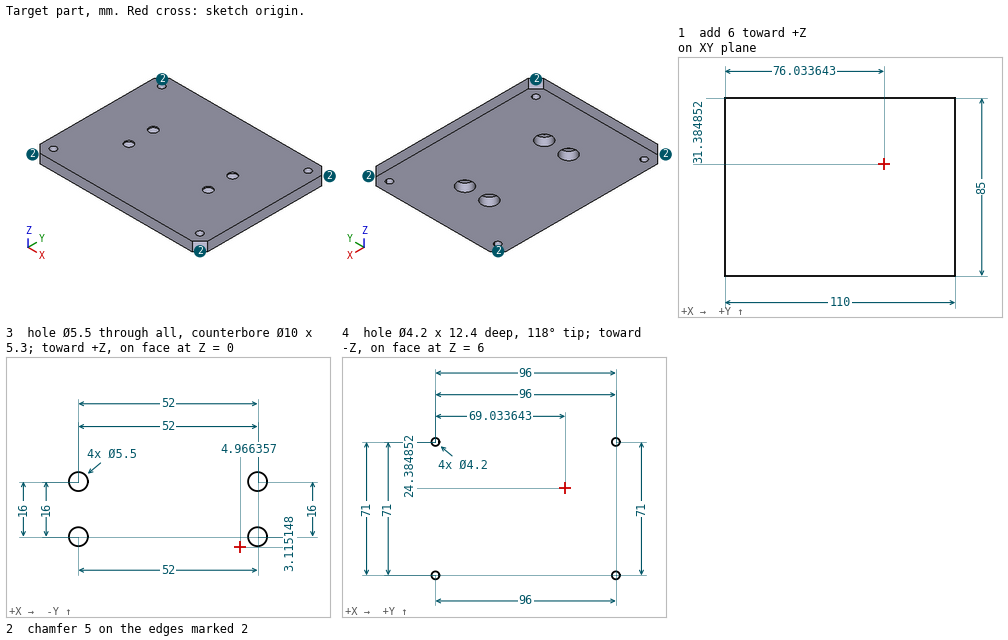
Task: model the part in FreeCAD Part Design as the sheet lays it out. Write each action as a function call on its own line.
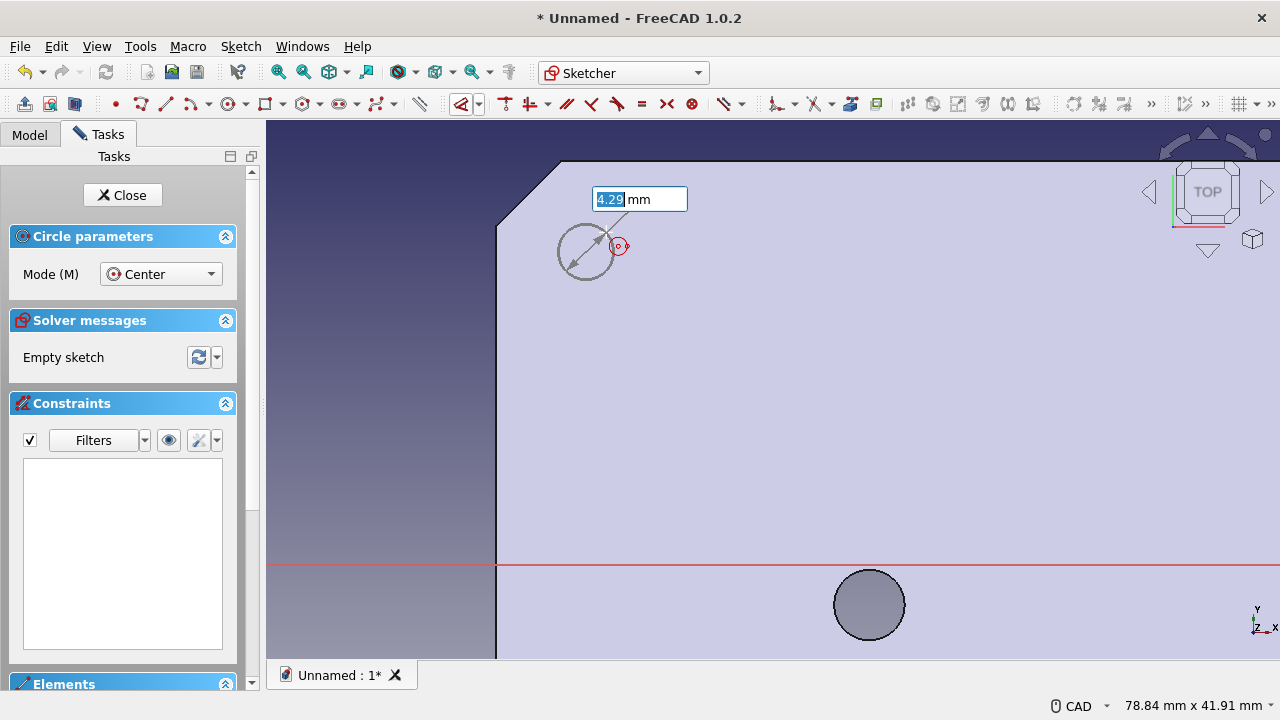
text(4.2)
key(Return)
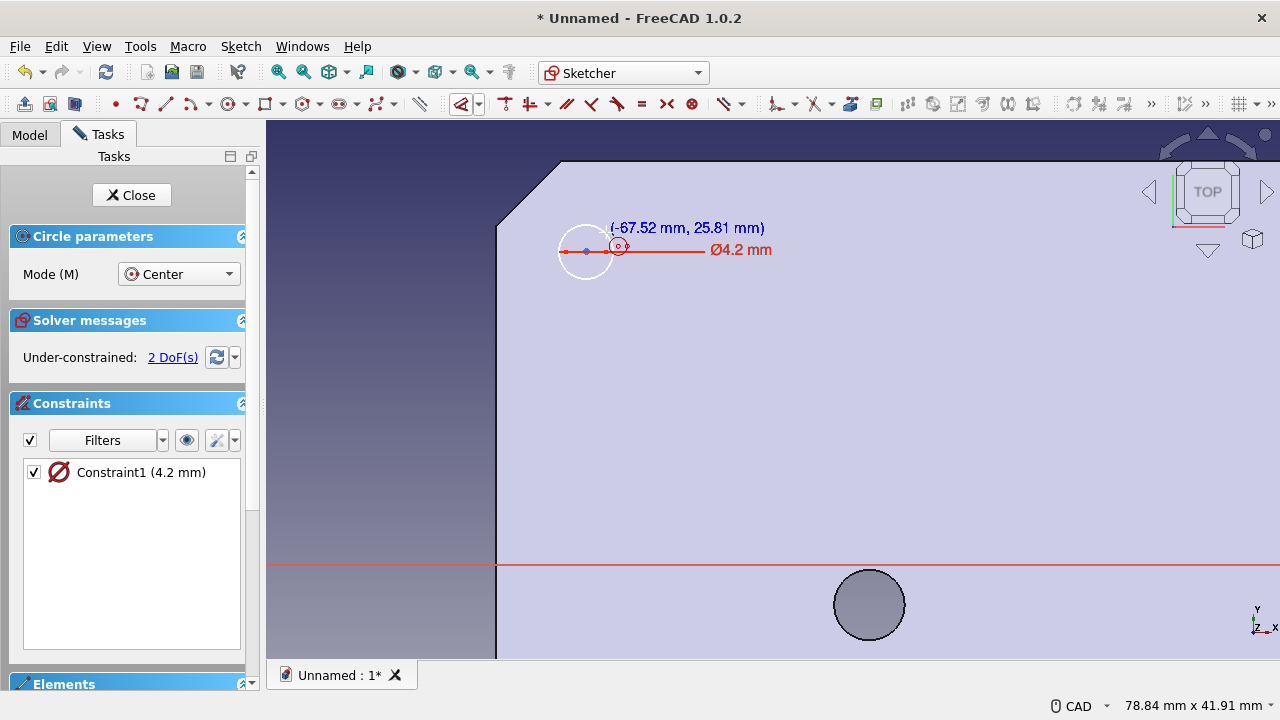
scroll(414, 204, down, 5)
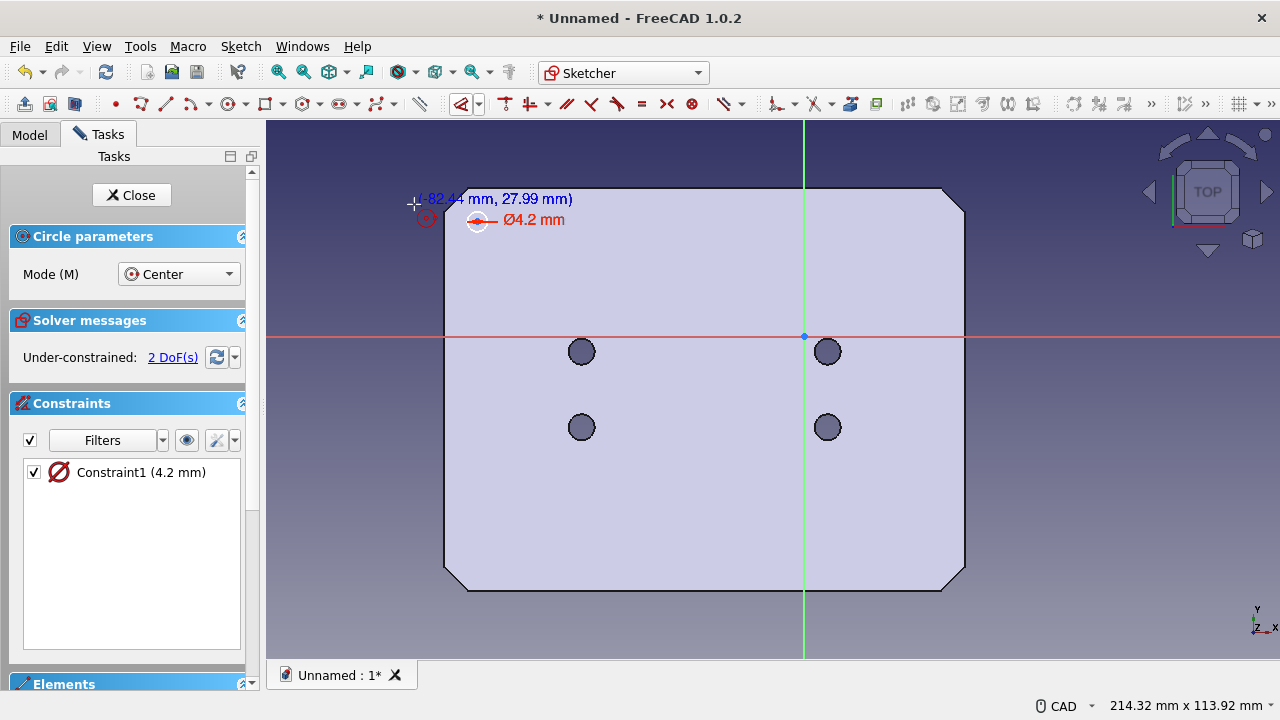
scroll(932, 222, up, 5)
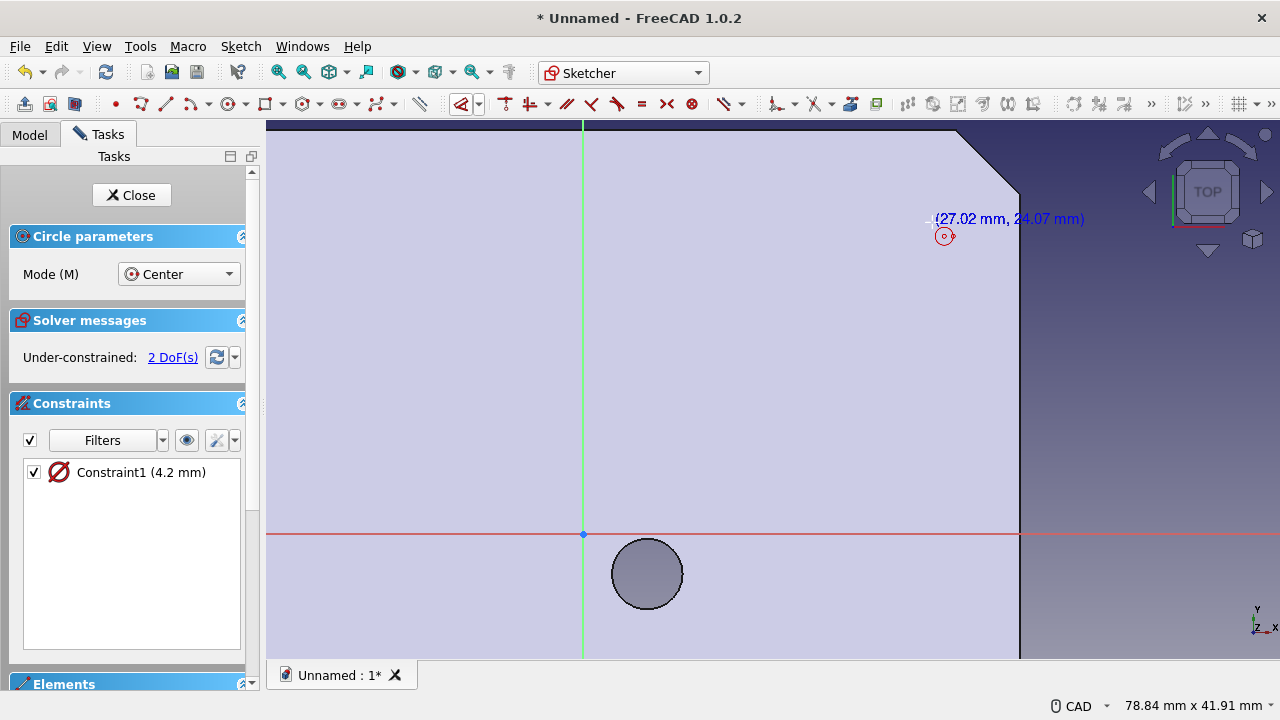
click(930, 220)
move(949, 201)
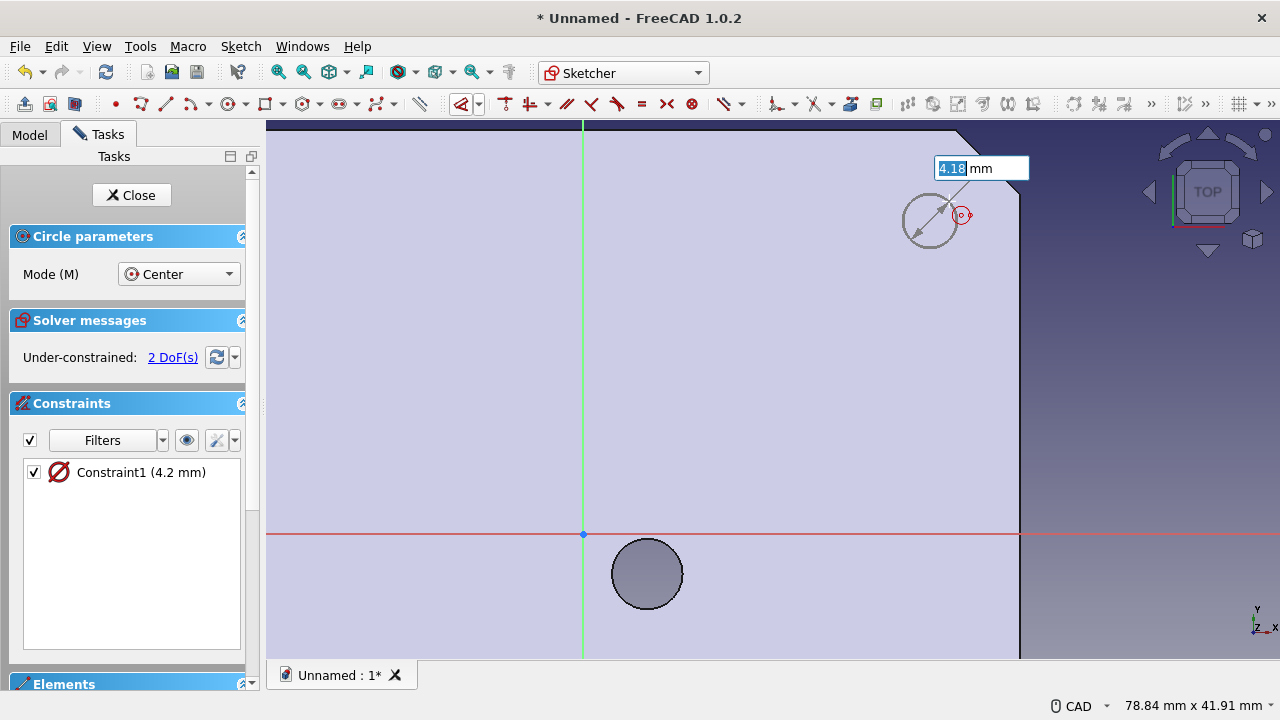
text(4.2)
key(Return)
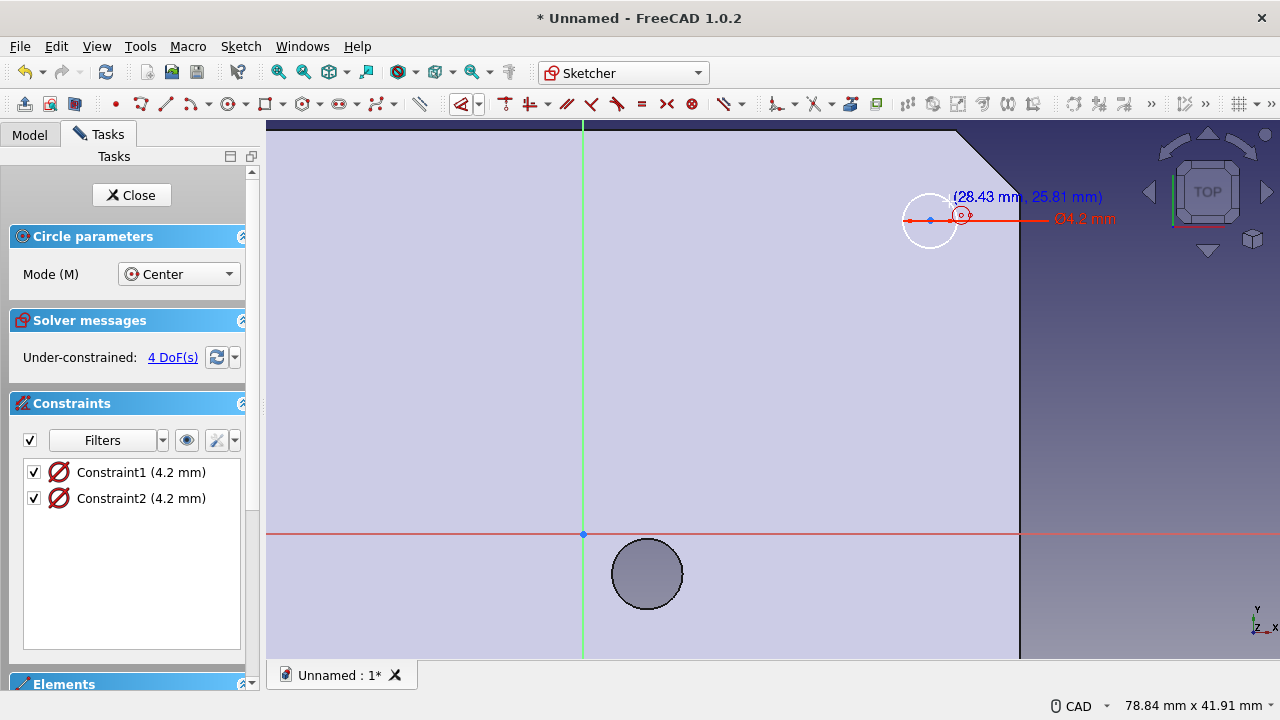
scroll(932, 222, down, 5)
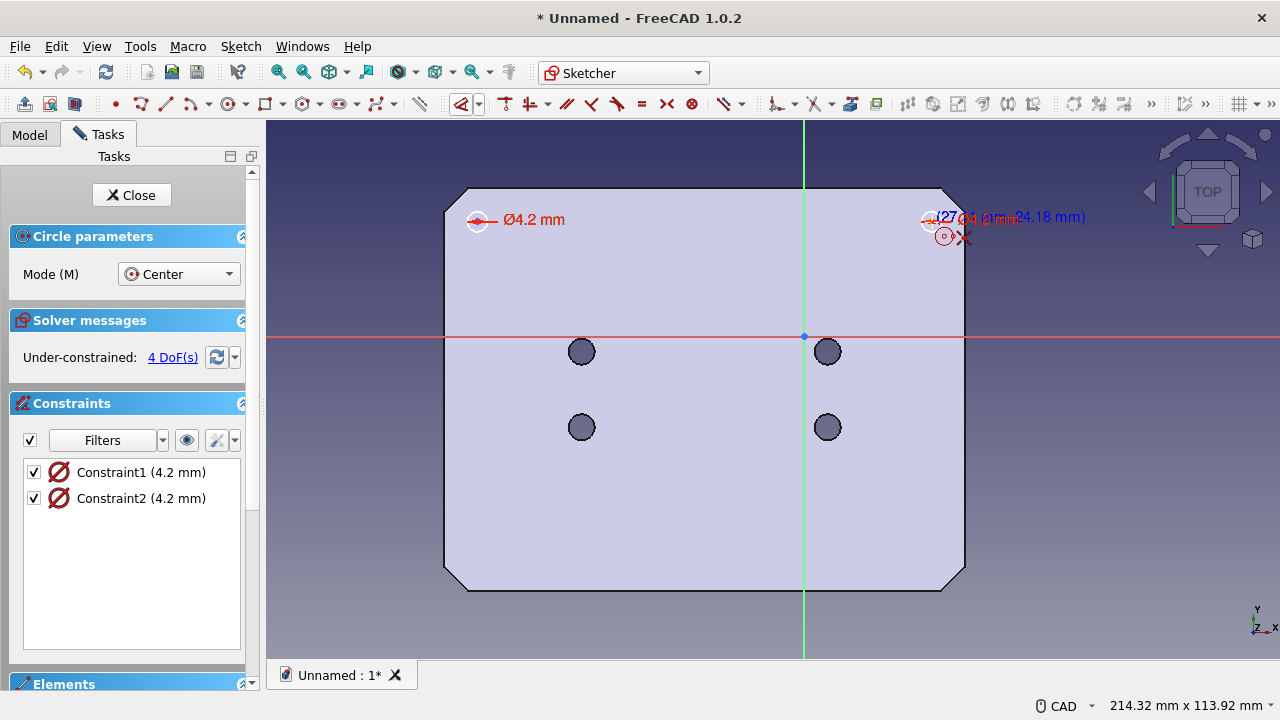
scroll(932, 557, up, 5)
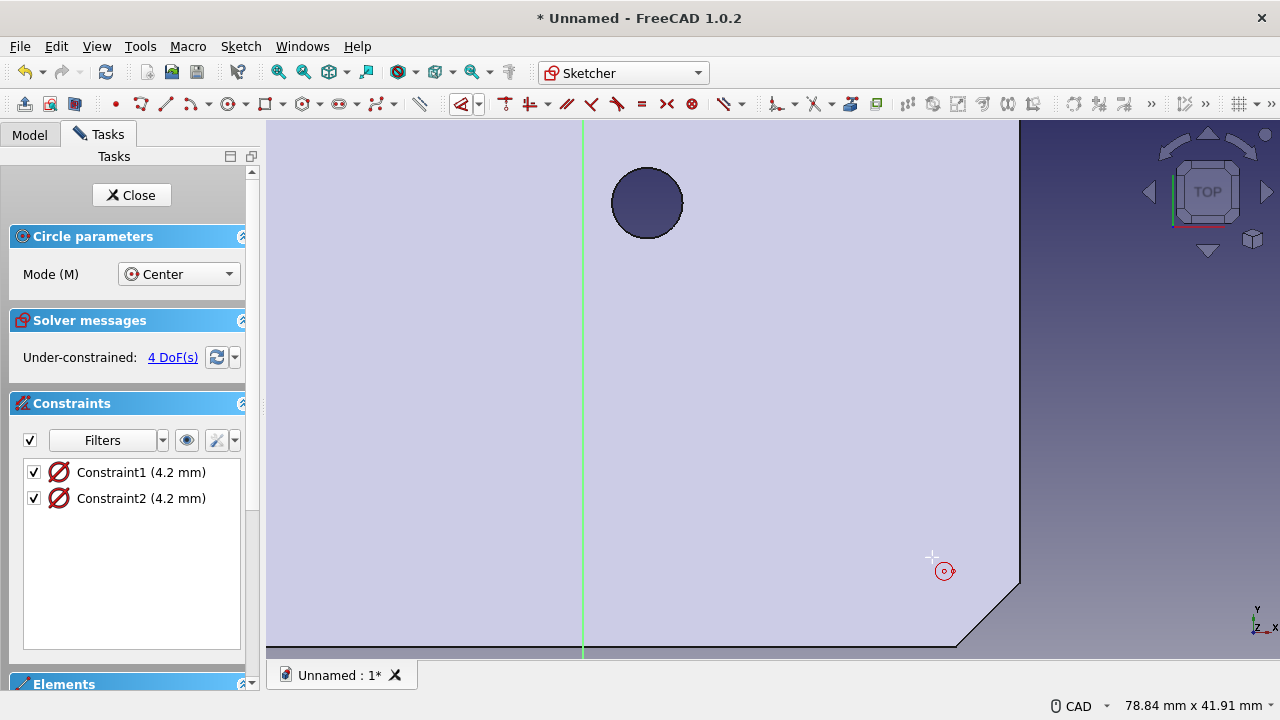
click(930, 557)
move(949, 538)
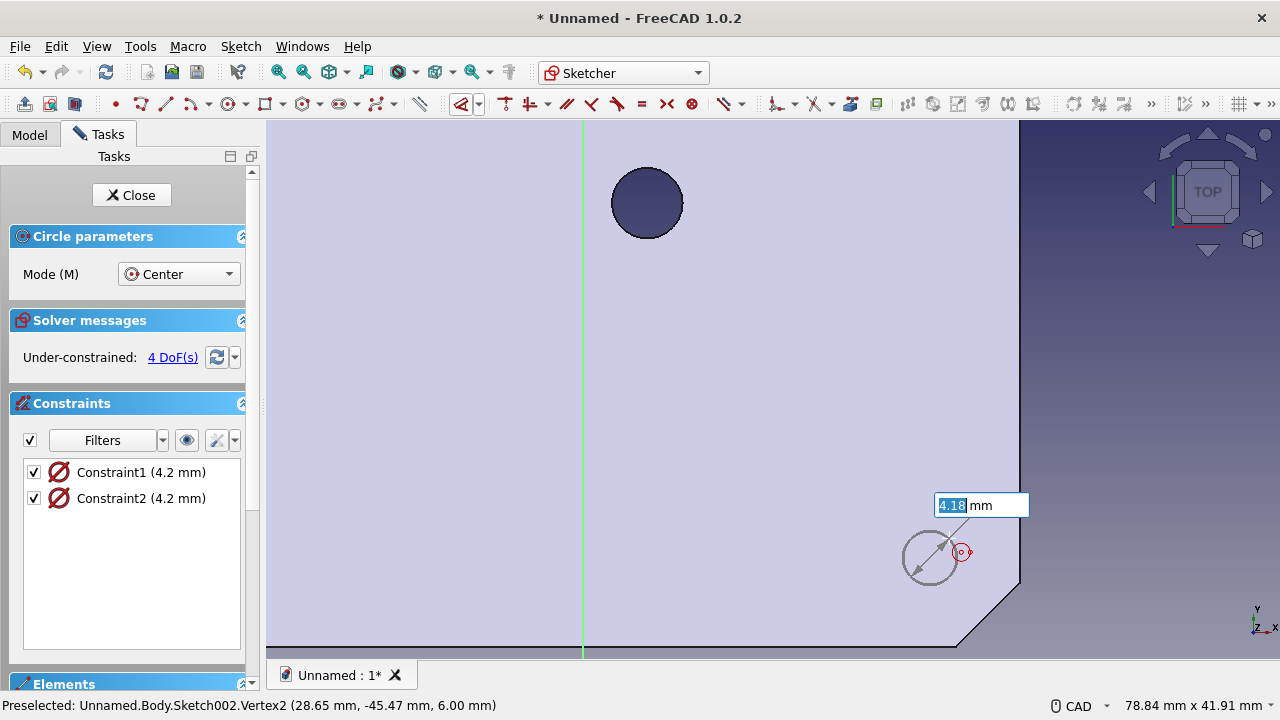
text(4.2)
key(Return)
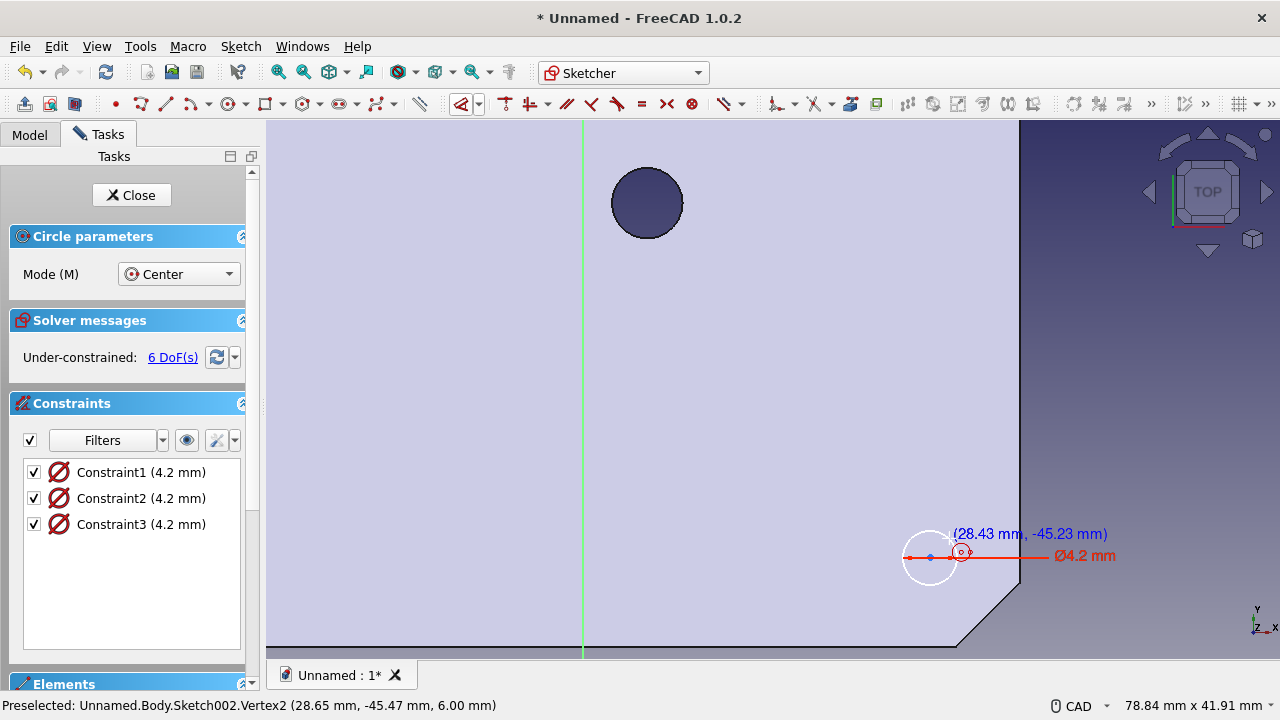
scroll(932, 558, down, 5)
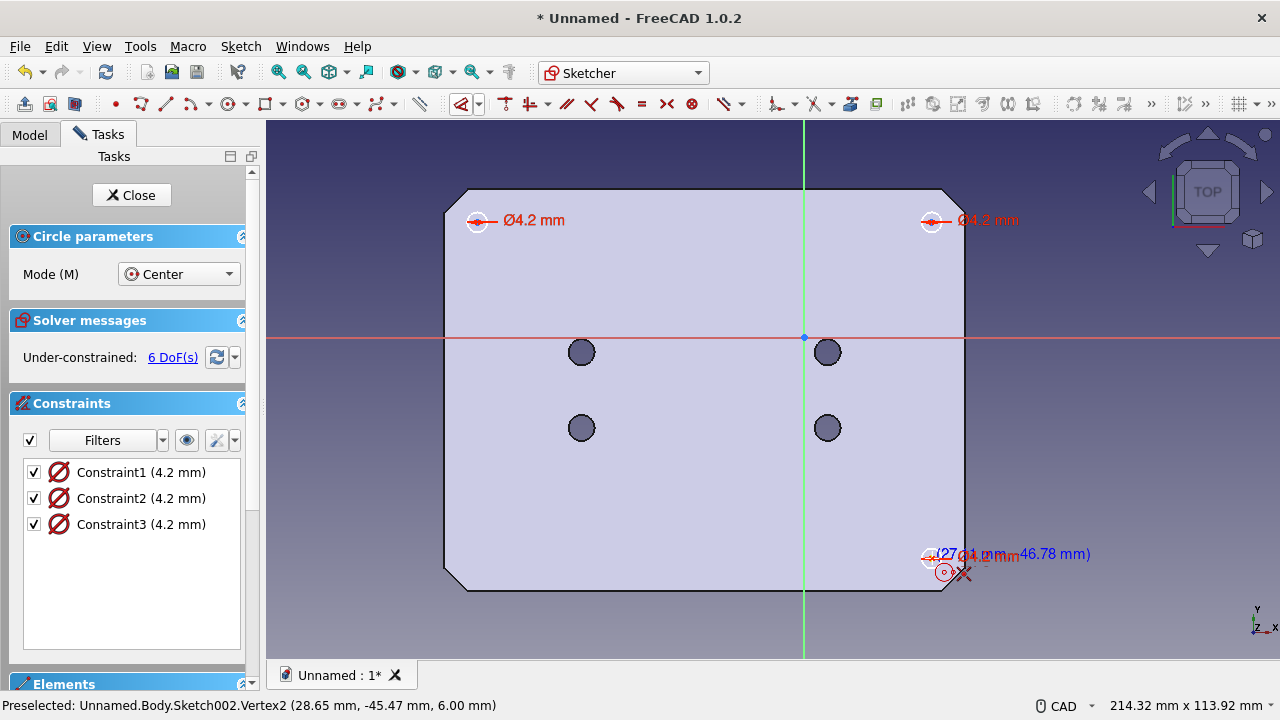
scroll(478, 558, up, 5)